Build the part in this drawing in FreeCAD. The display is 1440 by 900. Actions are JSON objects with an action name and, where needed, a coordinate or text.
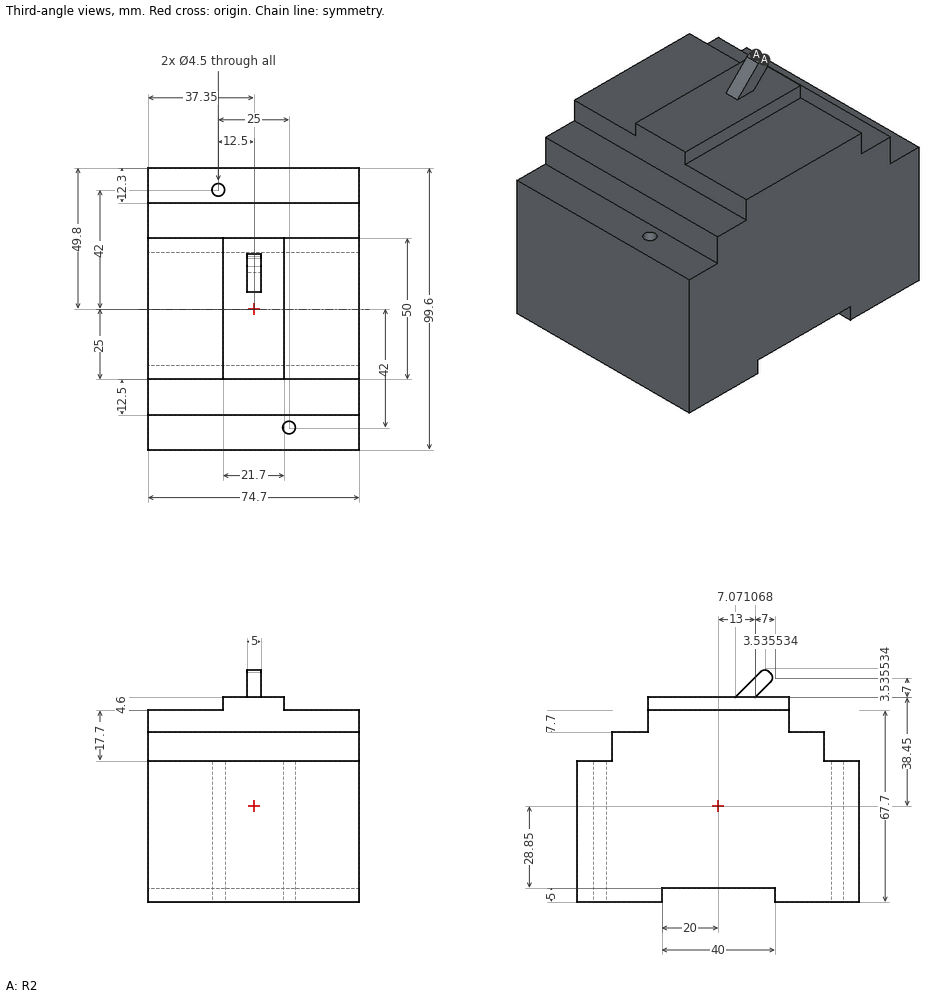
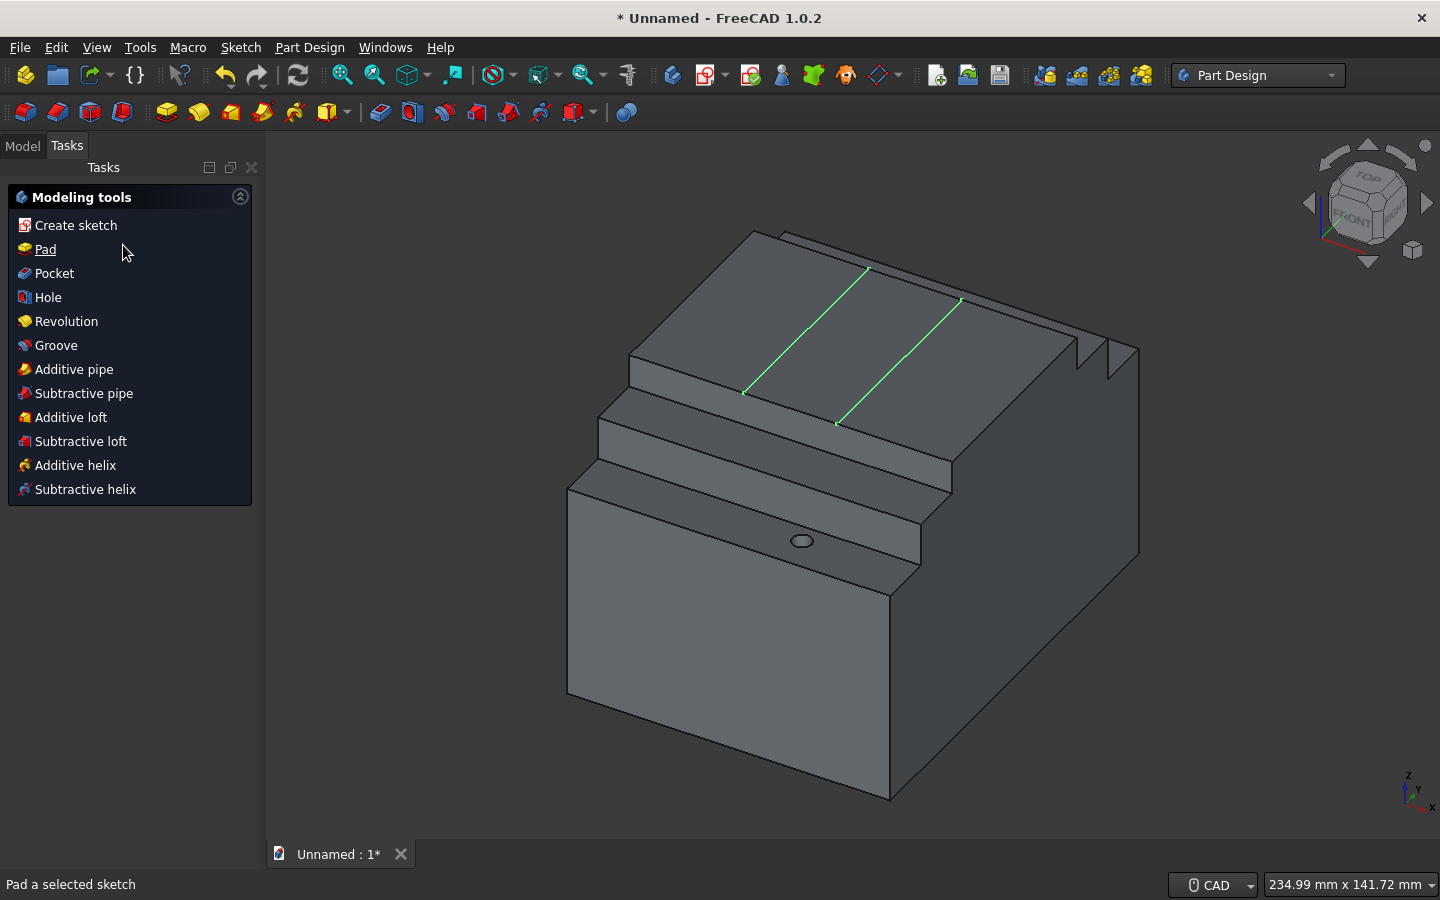
{"action": "left_click", "coordinate": [168, 112]}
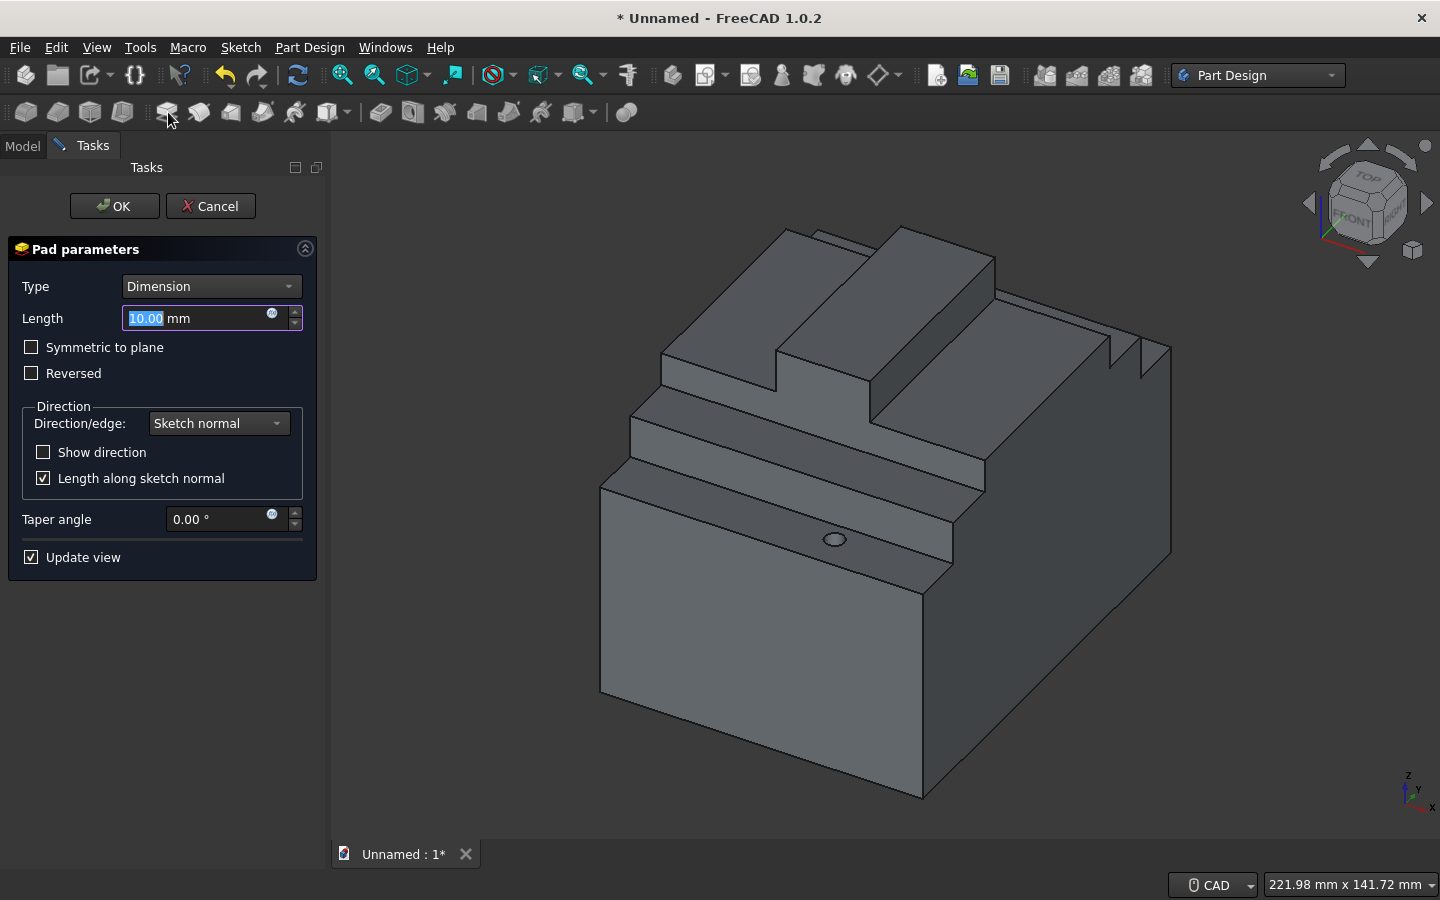
{"action": "type", "text": "4.6"}
{"action": "key", "text": "Tab"}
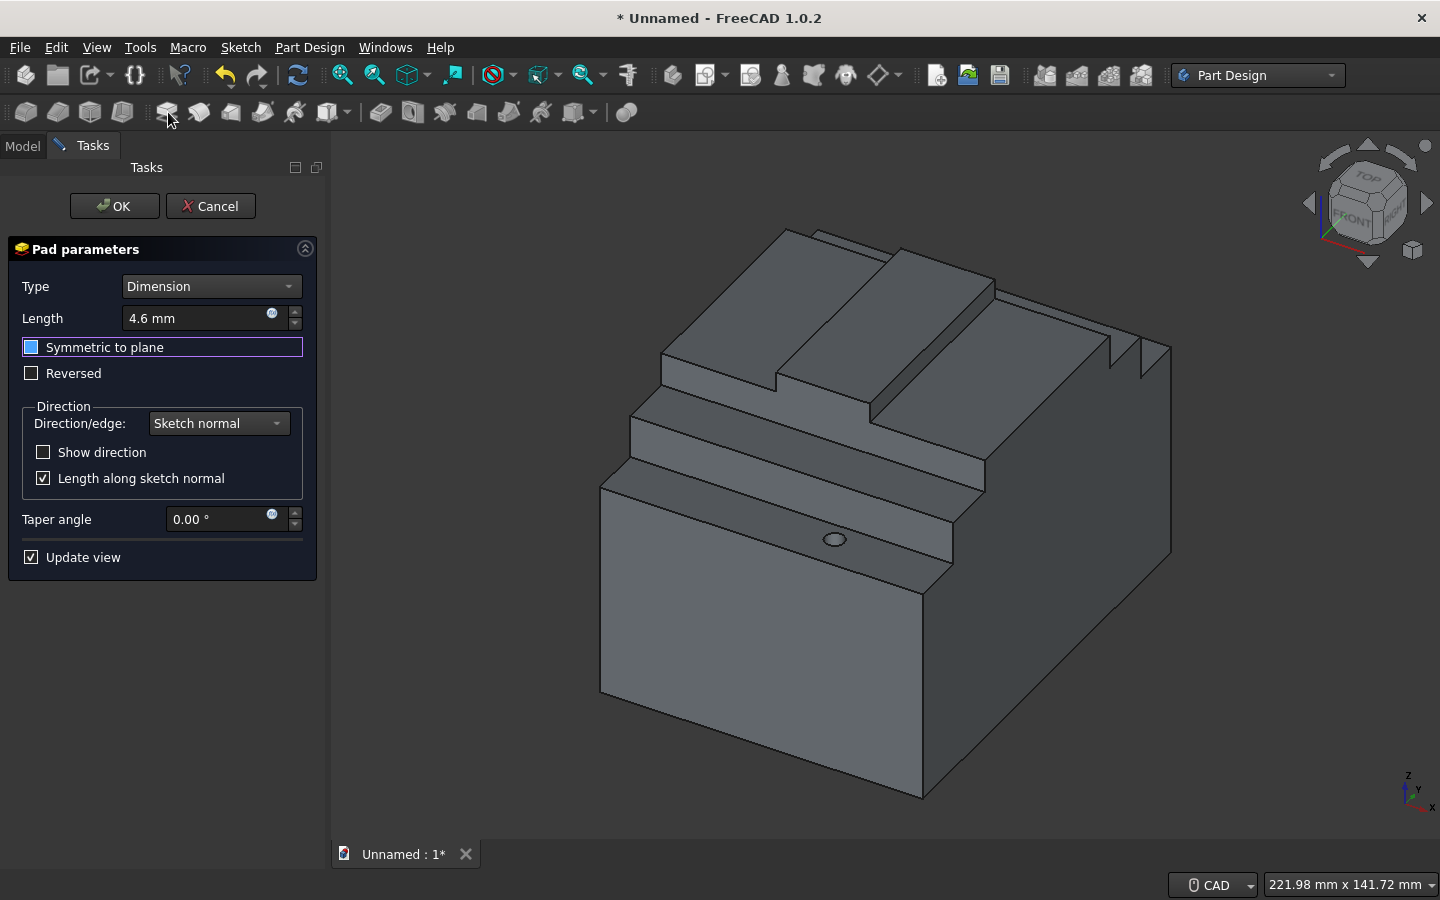
{"action": "left_click", "coordinate": [115, 206]}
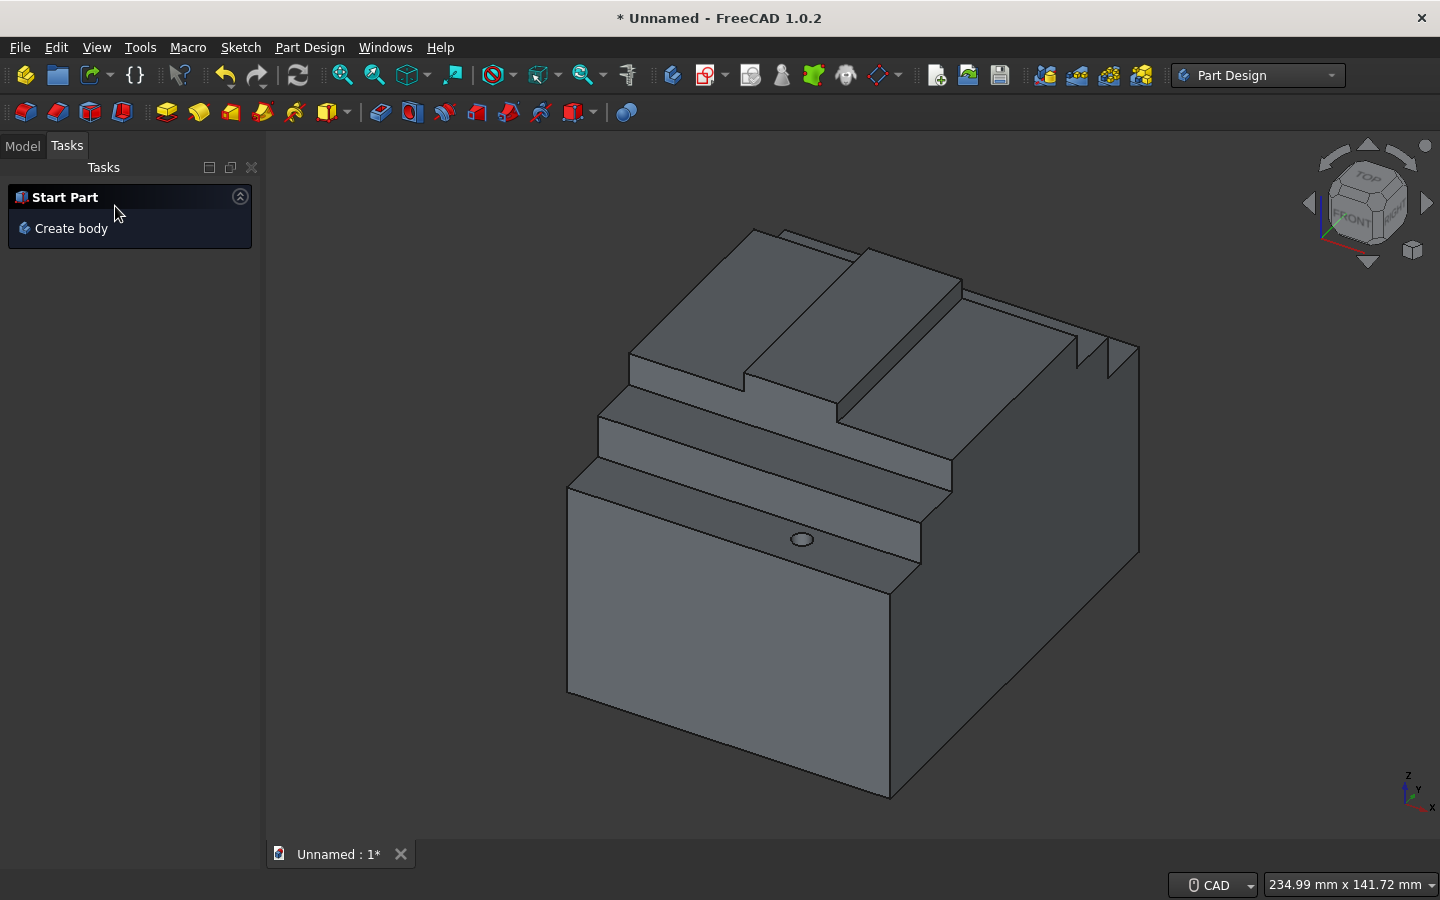
{"action": "left_click", "coordinate": [1015, 536]}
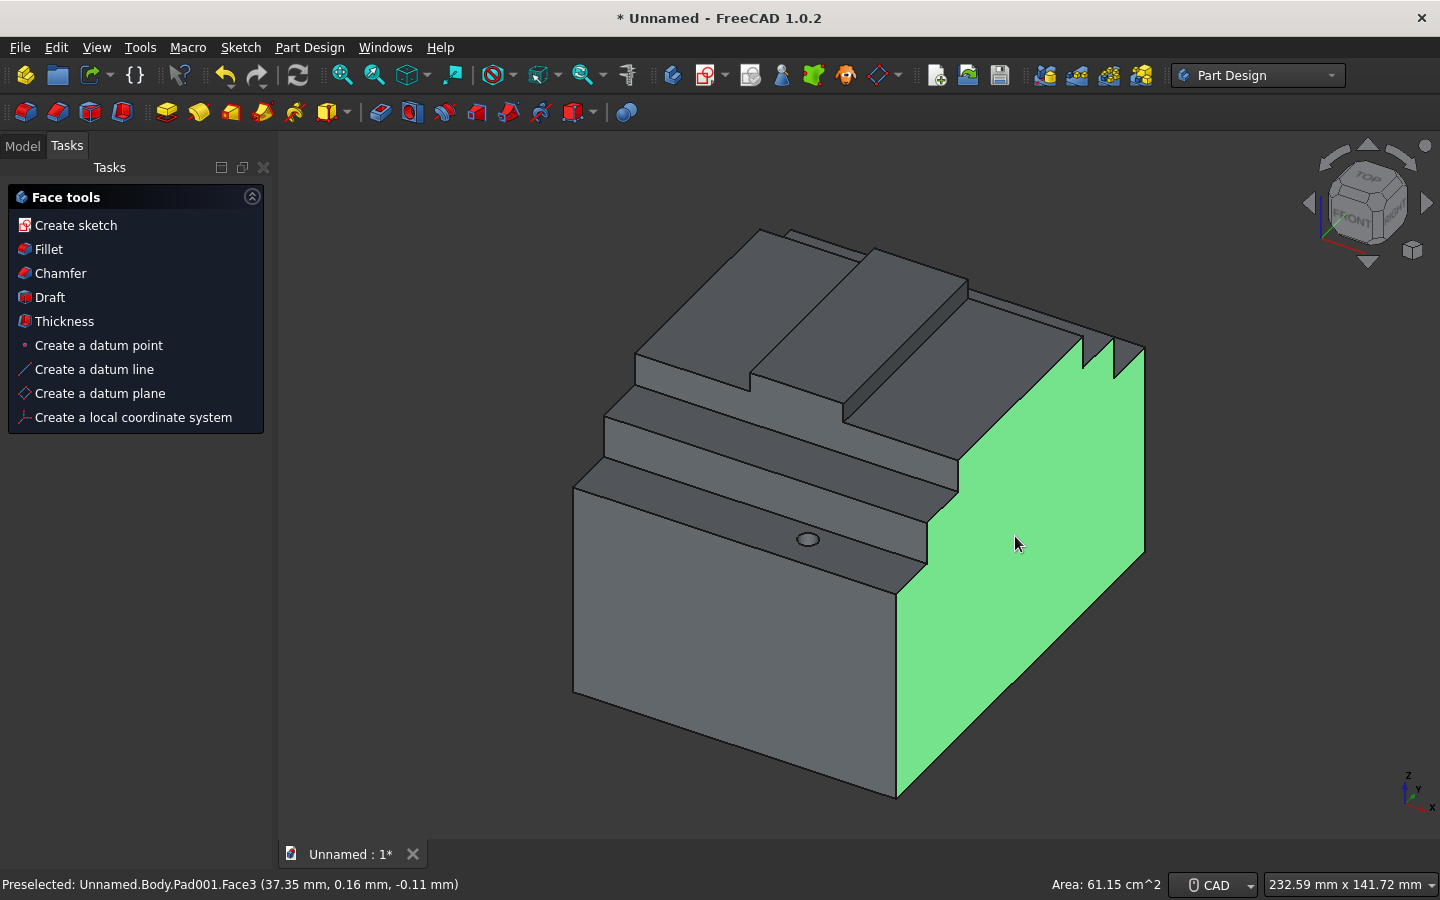
{"action": "left_click", "coordinate": [706, 76]}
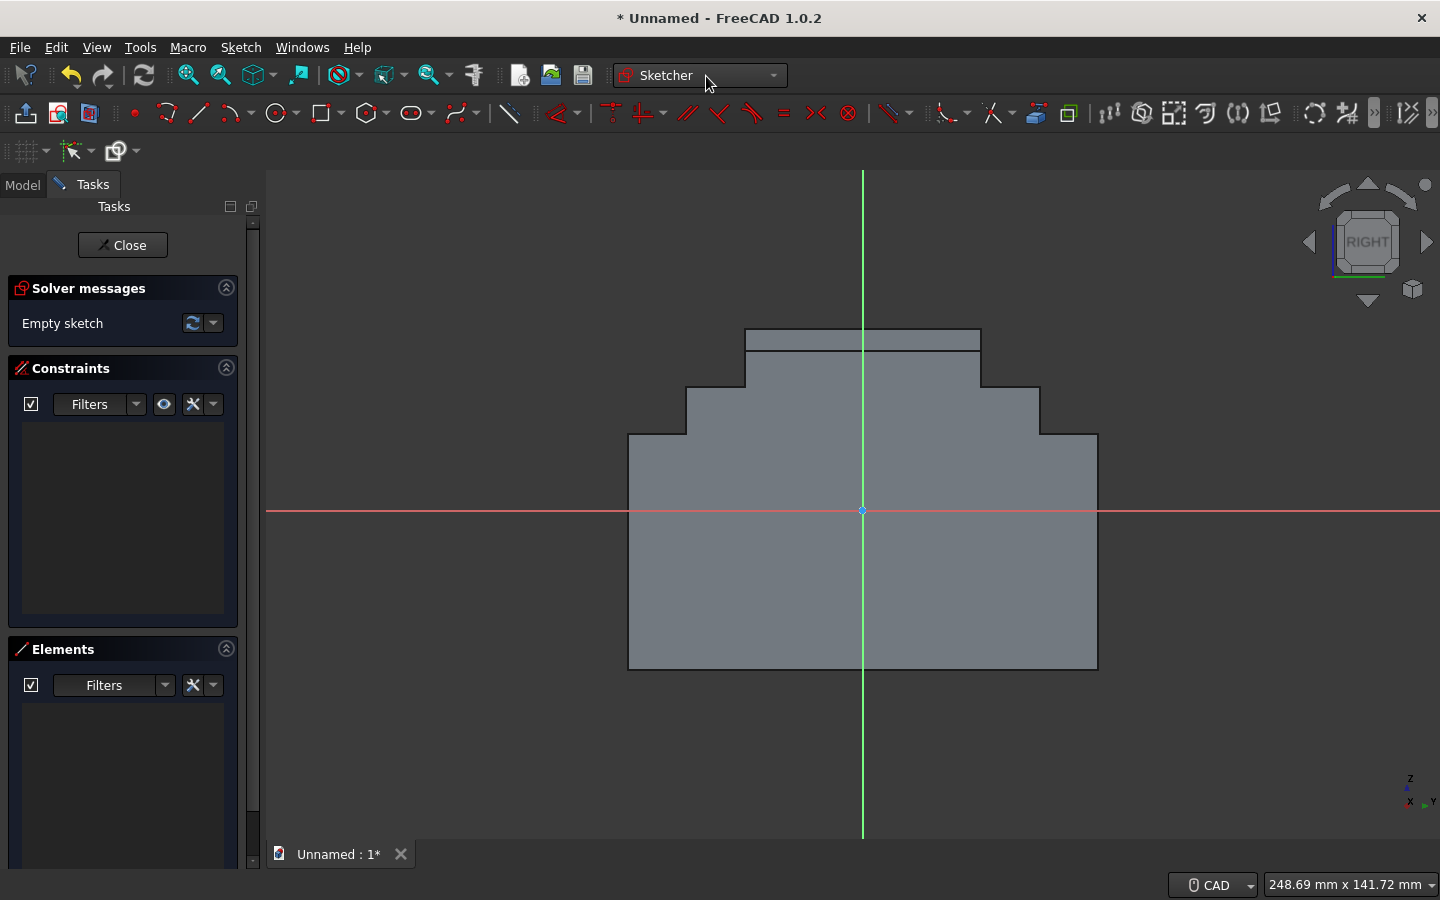
{"action": "scroll", "coordinate": [909, 641], "scroll_direction": "up", "scroll_amount": 5}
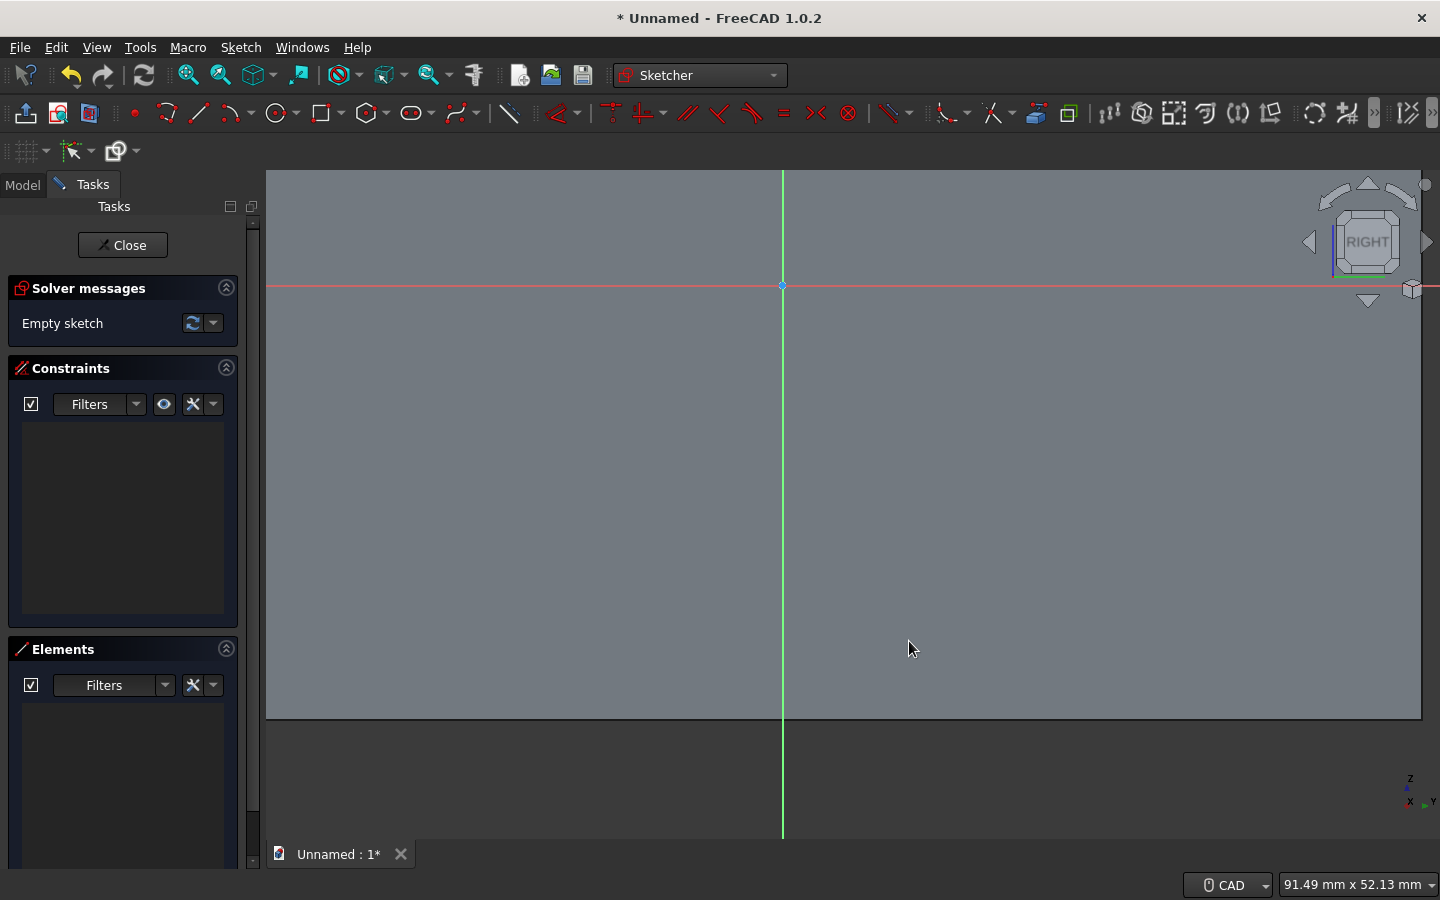
{"action": "left_click", "coordinate": [322, 114]}